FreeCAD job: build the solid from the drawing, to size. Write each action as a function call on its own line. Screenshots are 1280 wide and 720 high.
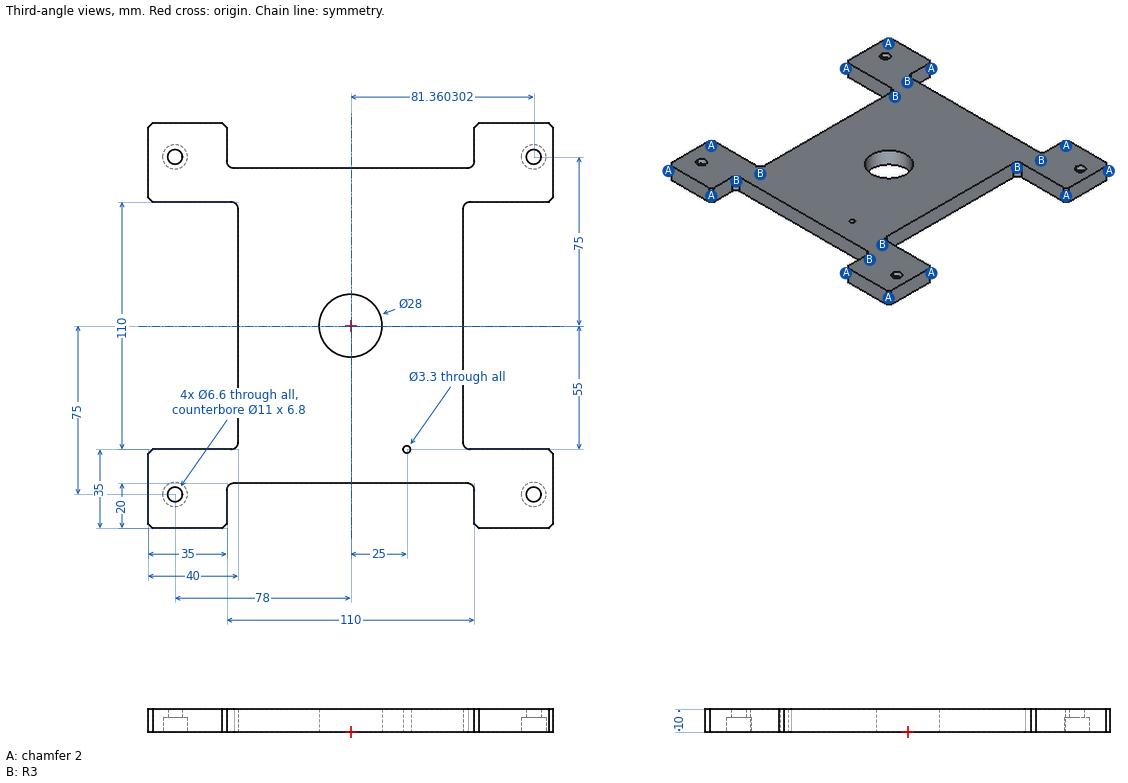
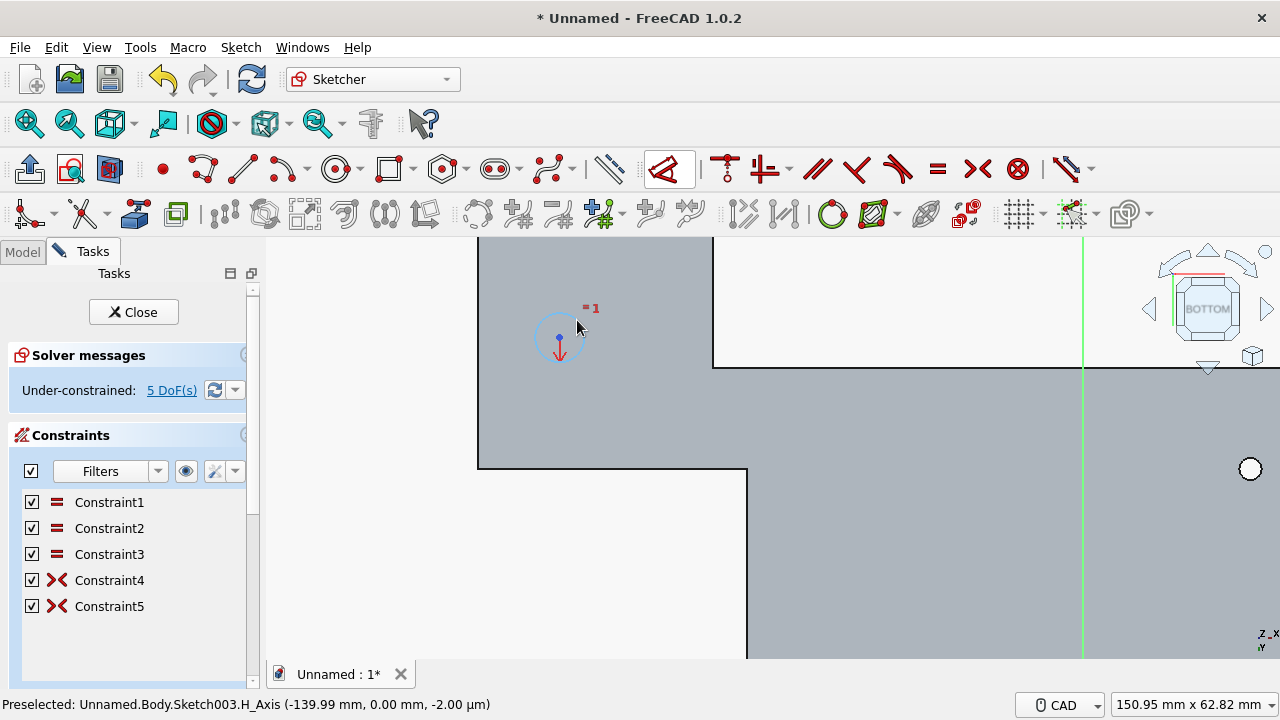
click(577, 320)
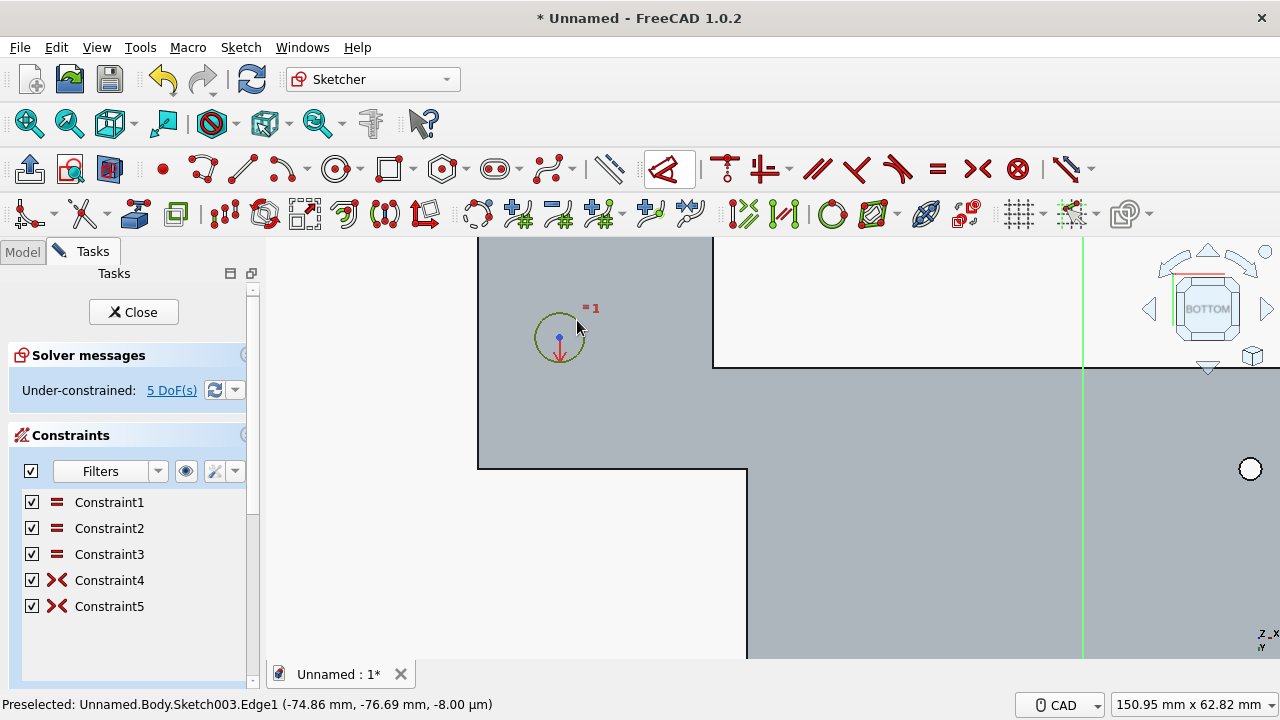
key(k)
key(o)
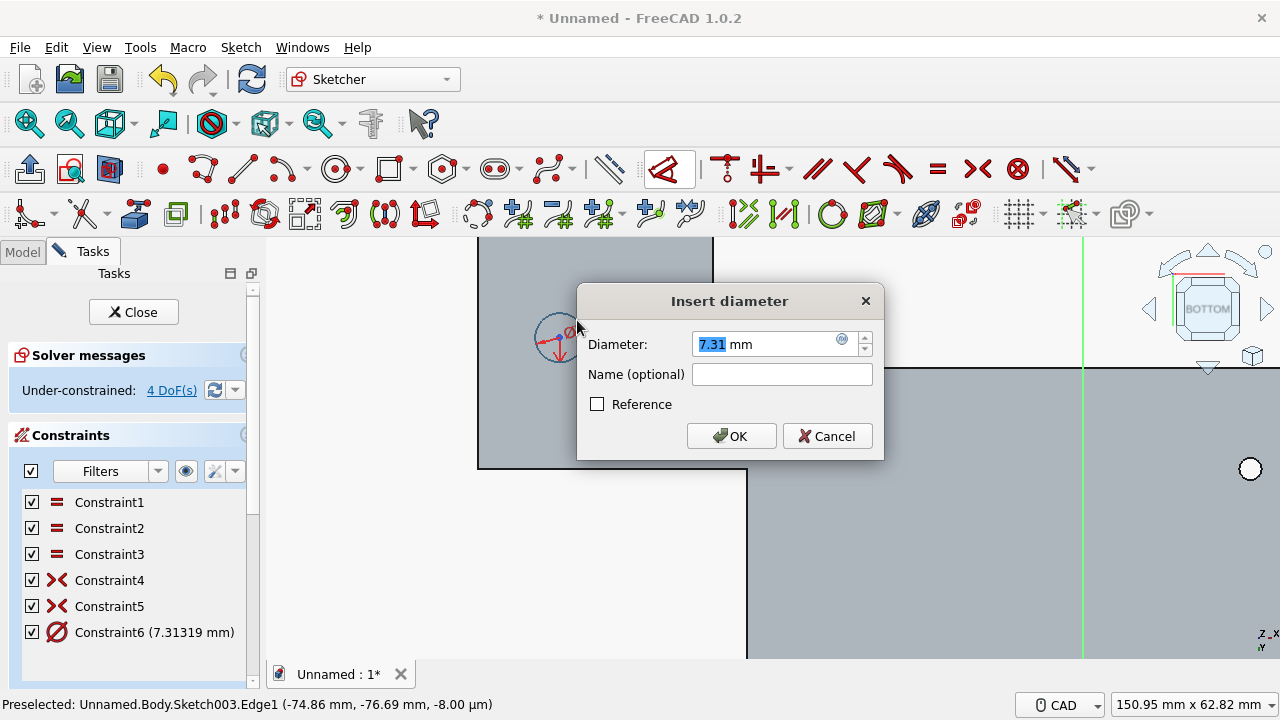
text(6.6)
key(Return)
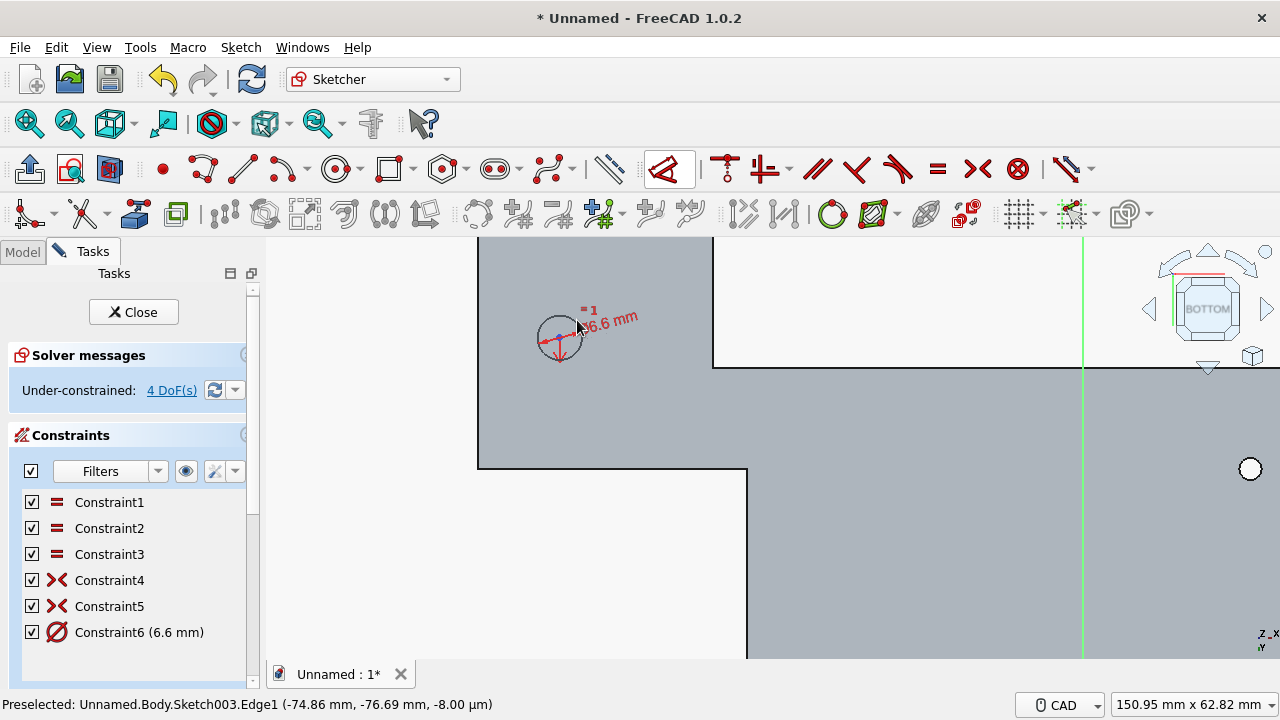
scroll(577, 320, down, 7)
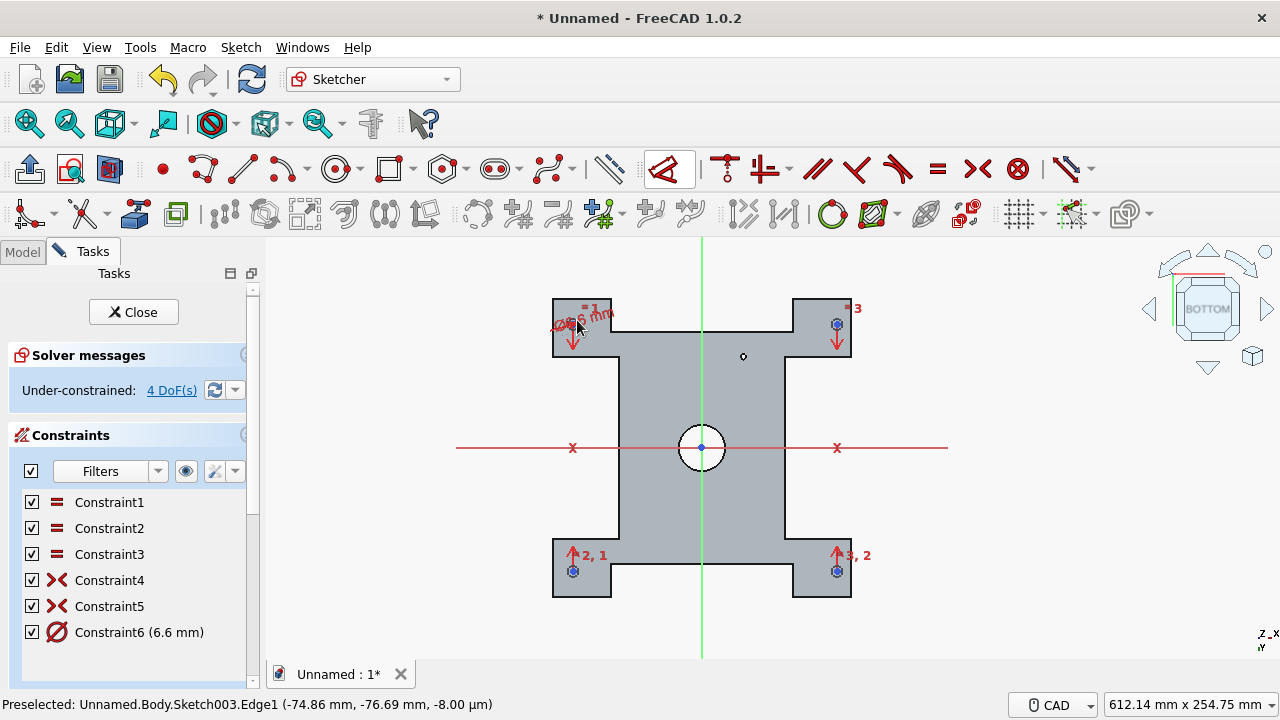
click(573, 325)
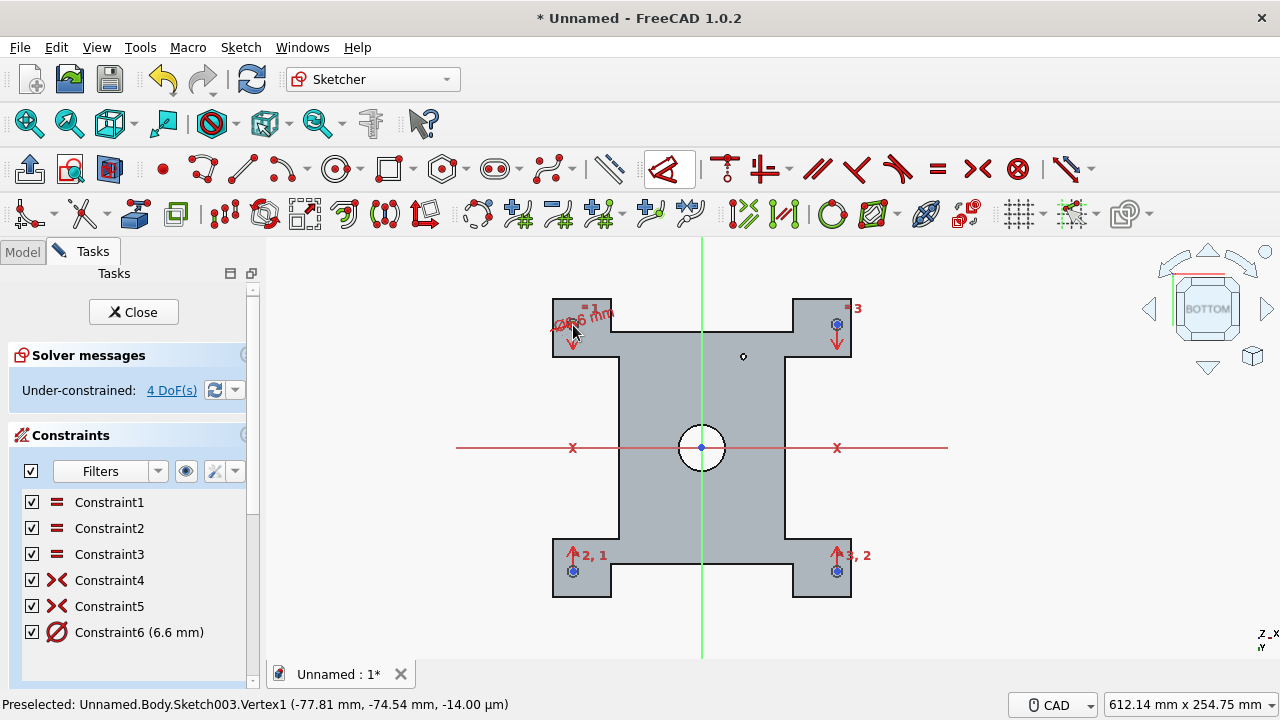
click(690, 170)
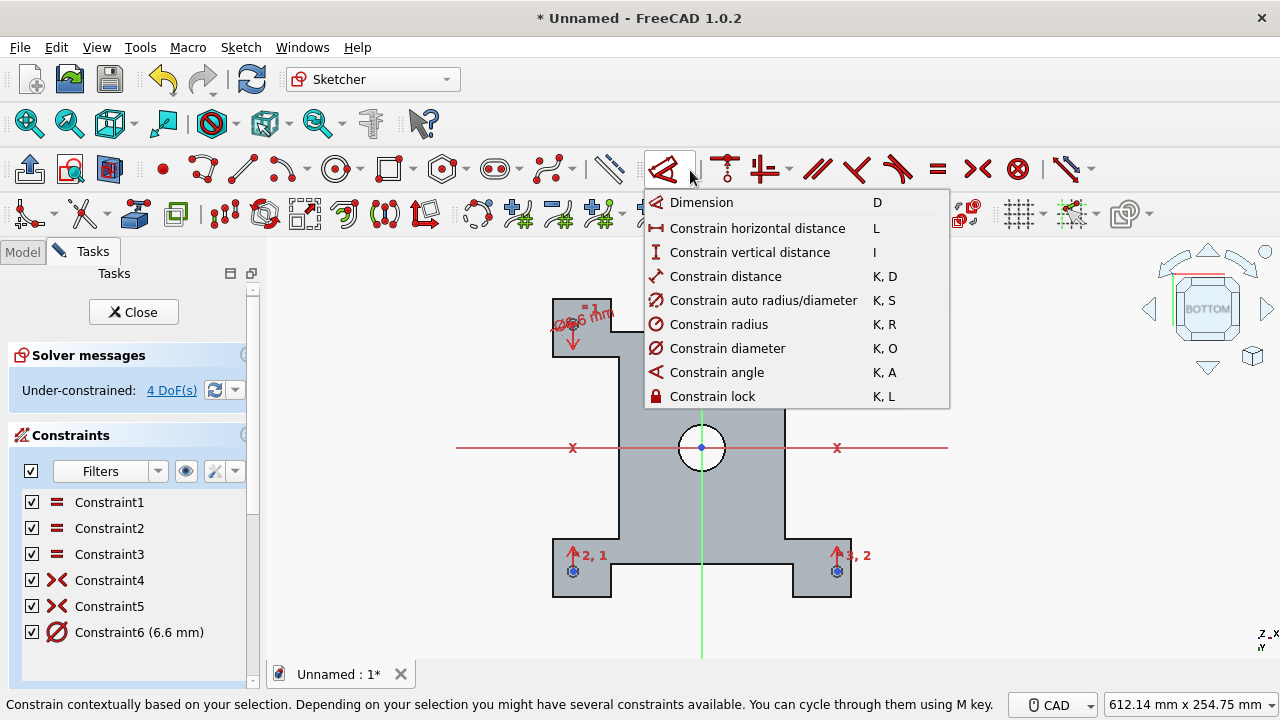
click(797, 228)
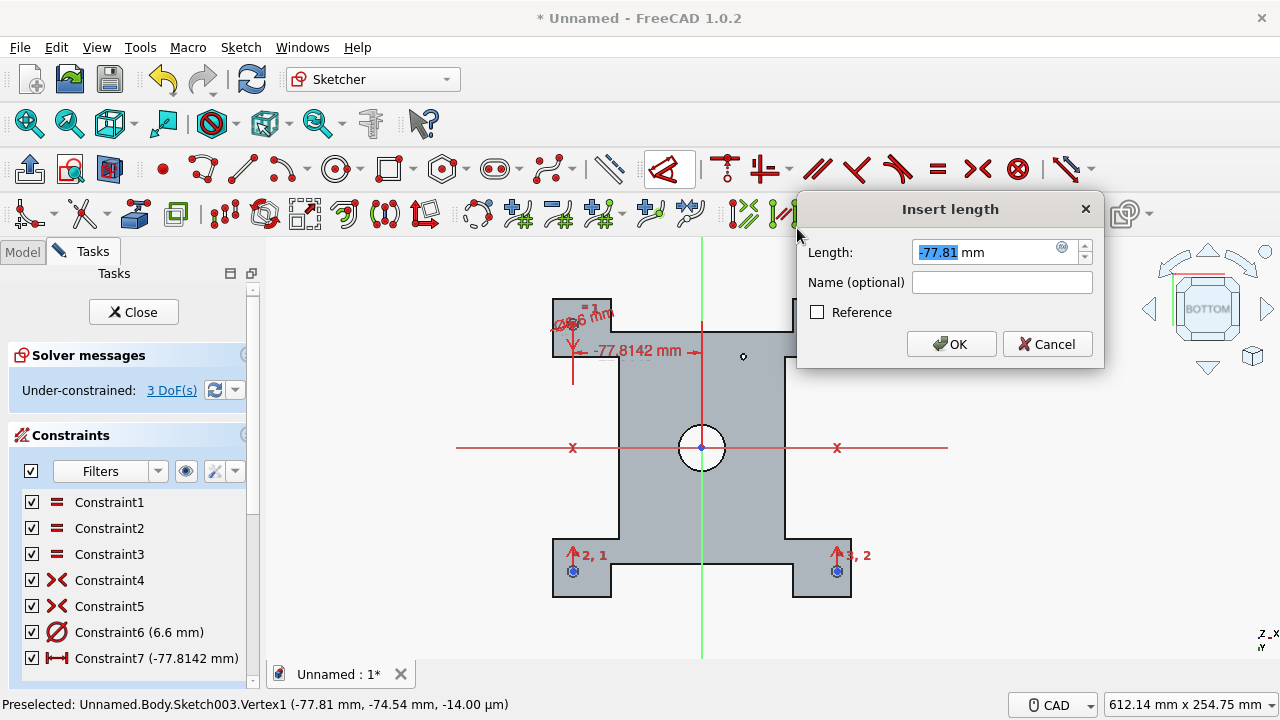
text(-78)
key(Return)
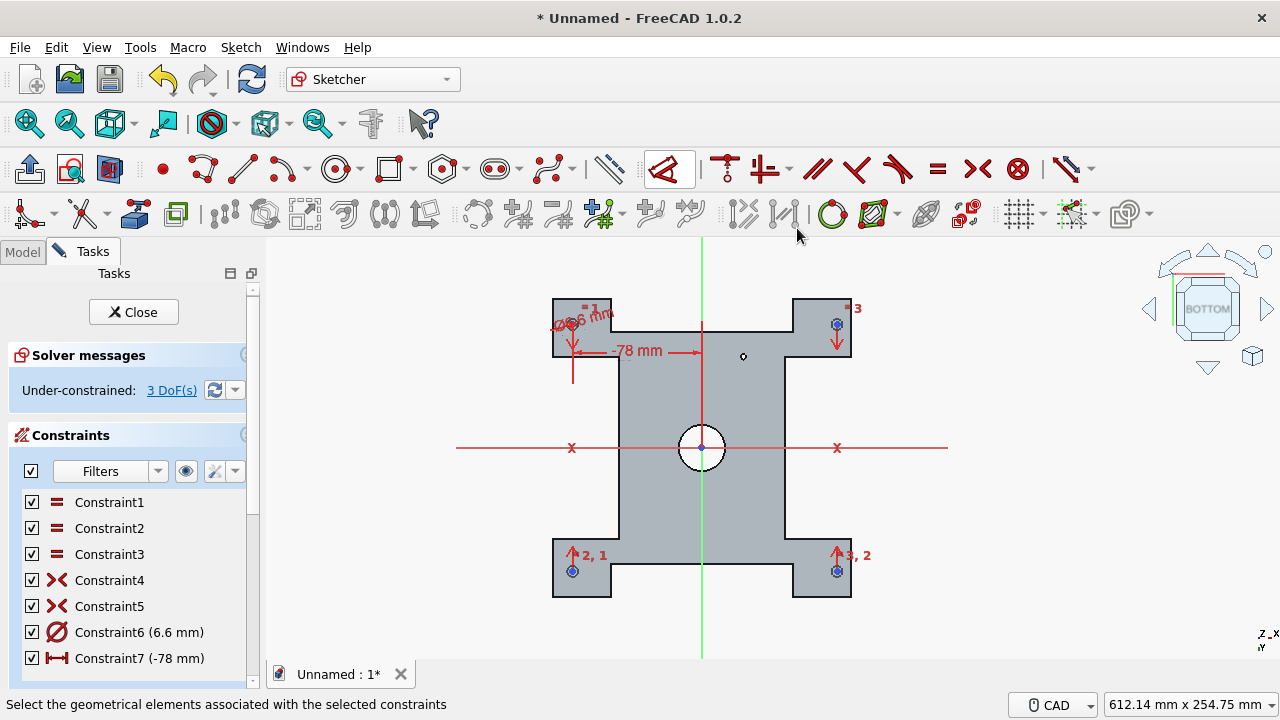
click(573, 325)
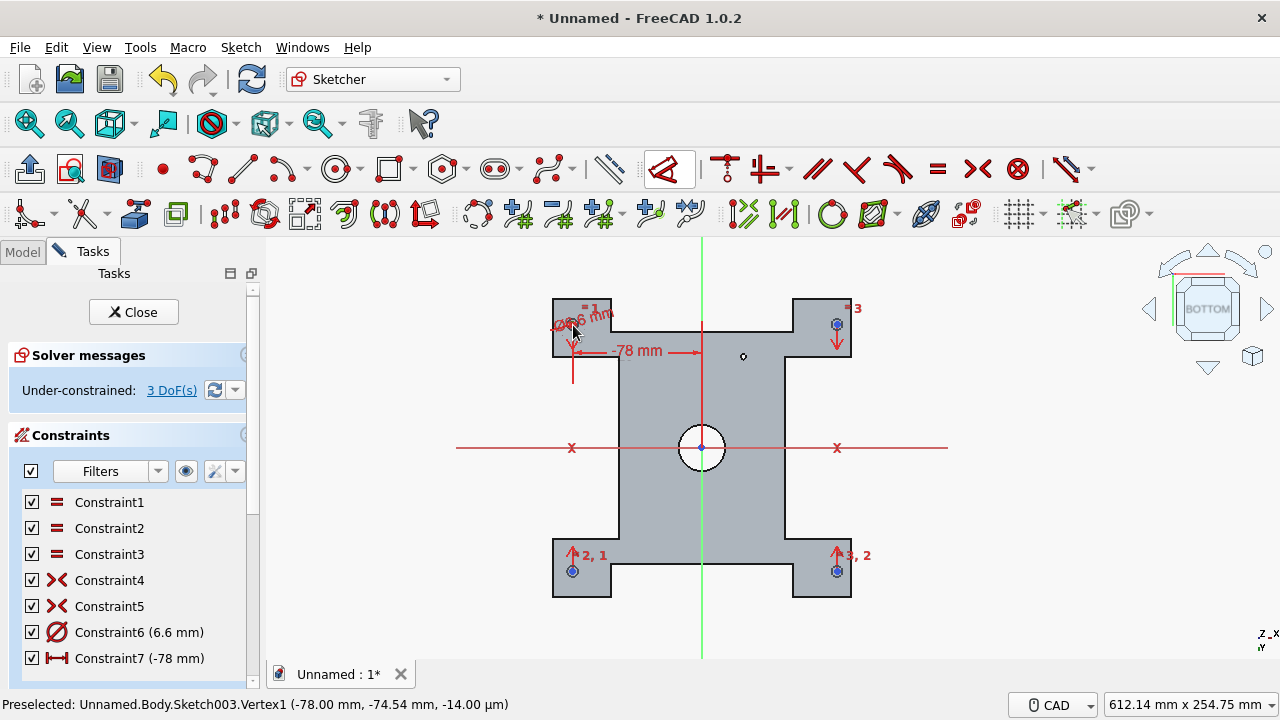
key(i)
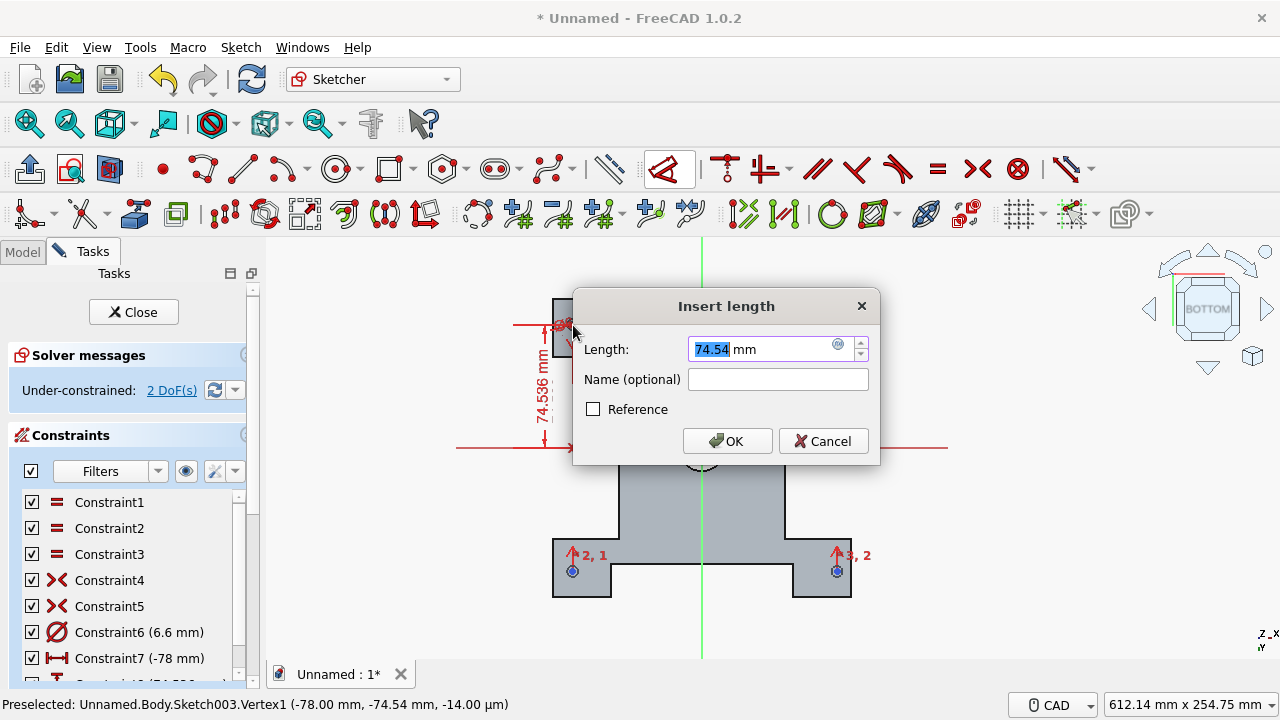
text(75)
key(Return)